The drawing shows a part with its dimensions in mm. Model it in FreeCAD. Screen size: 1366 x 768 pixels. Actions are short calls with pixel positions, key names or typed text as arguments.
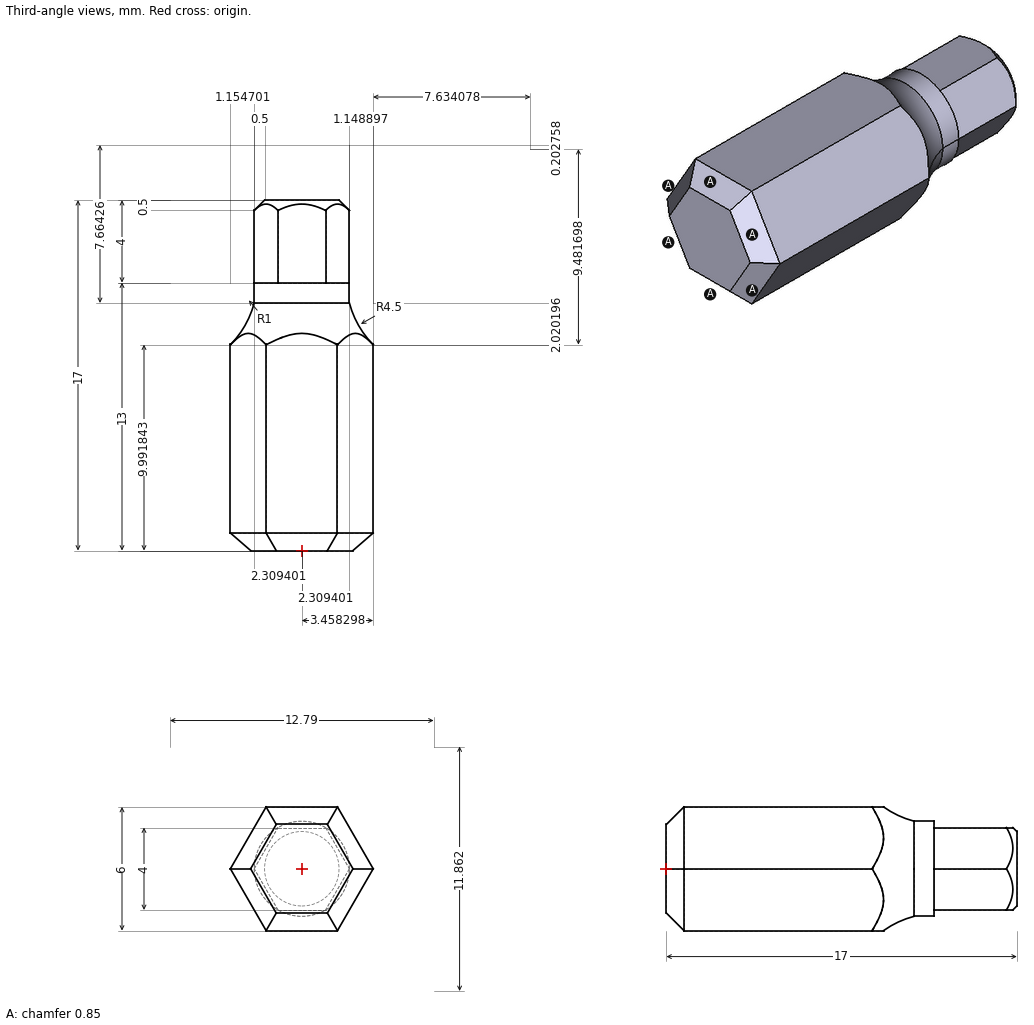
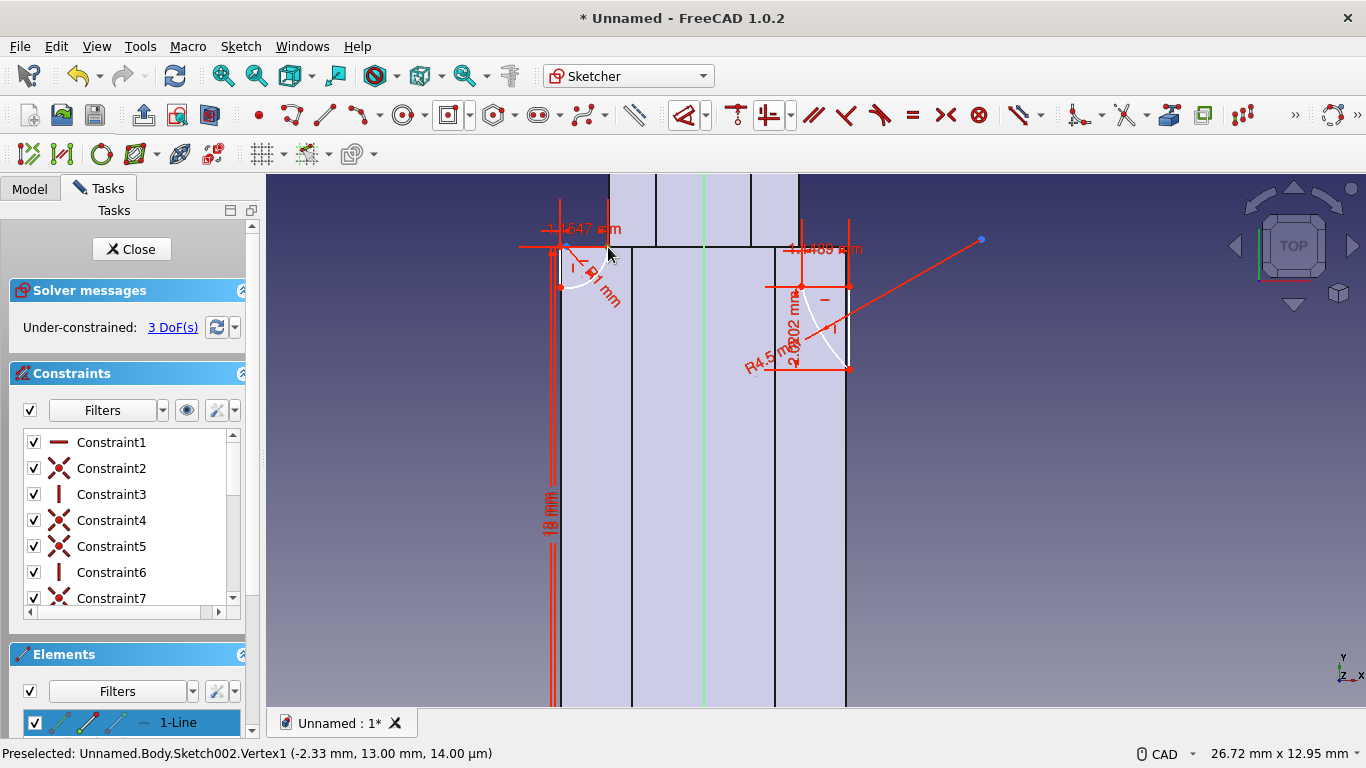
key(l)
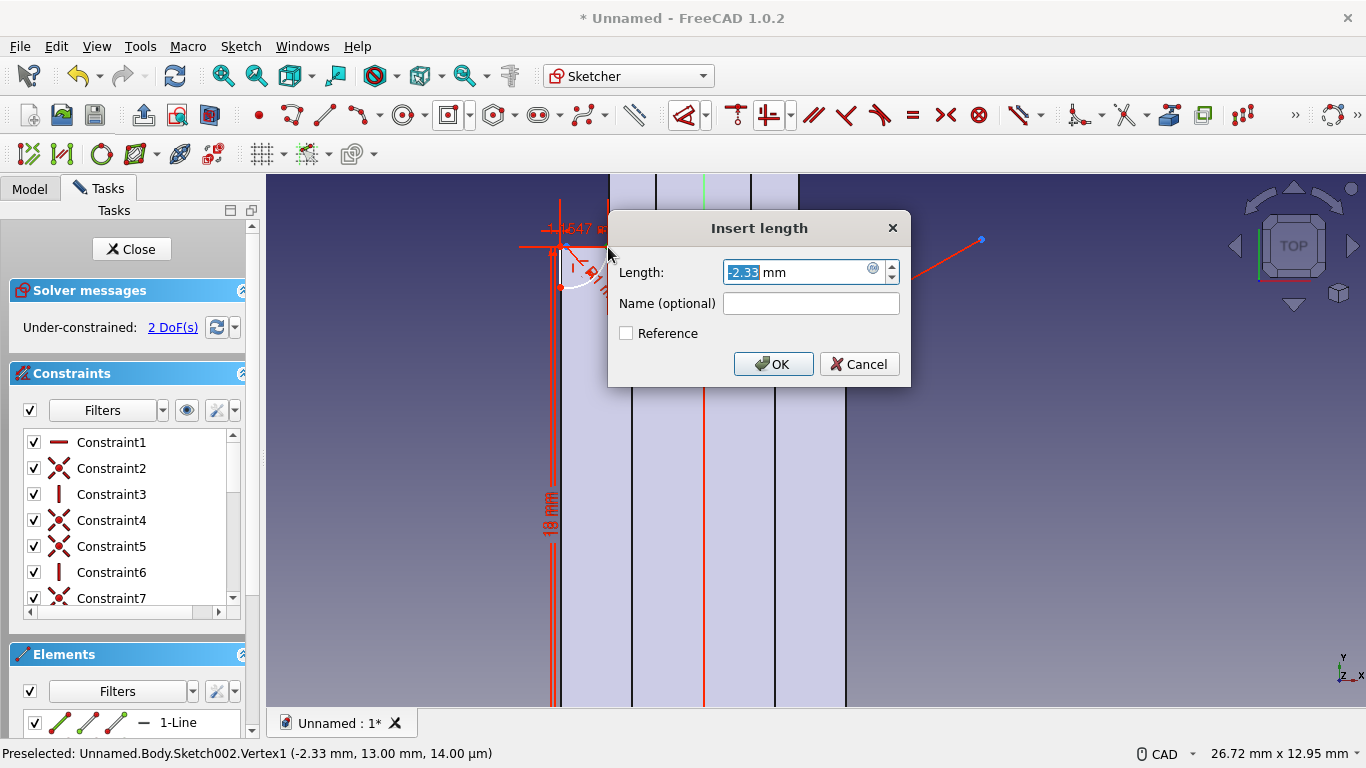
text(-2.309401)
key(Return)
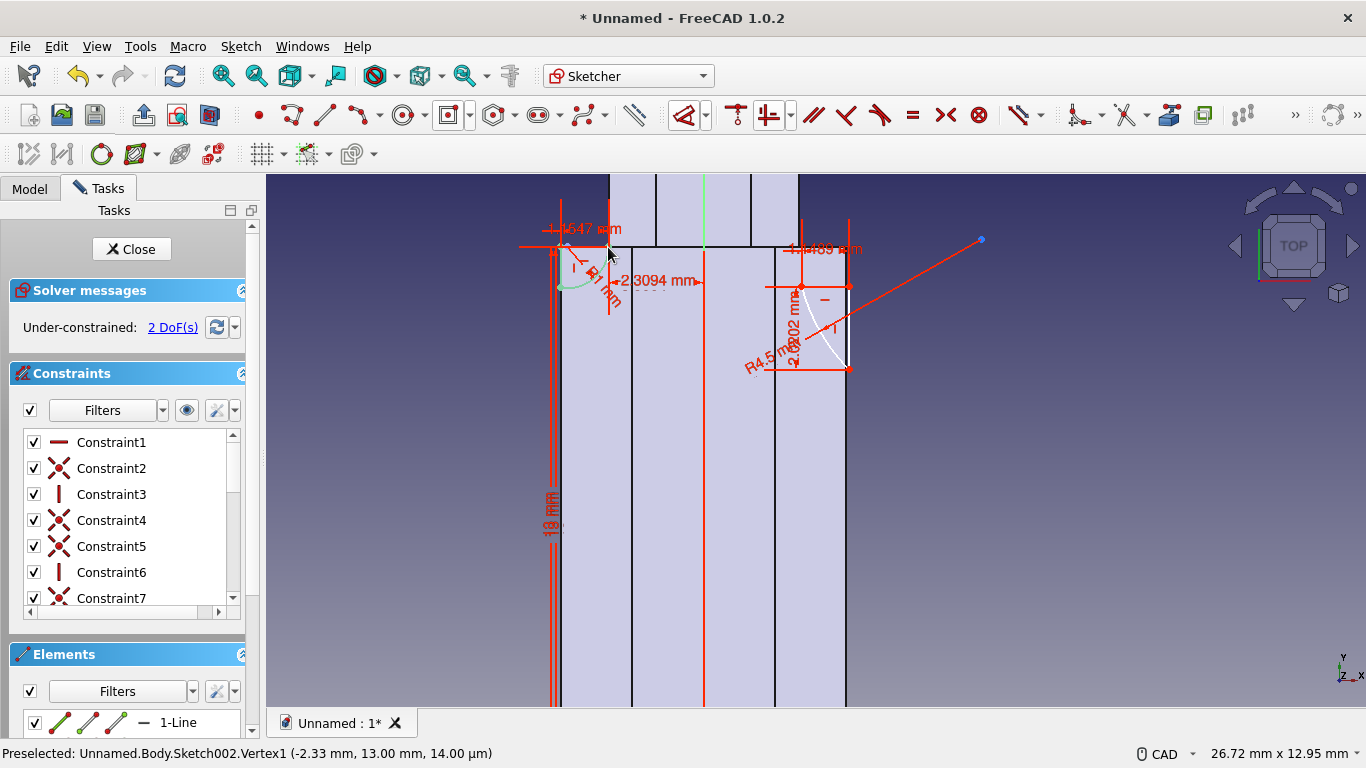
click(849, 370)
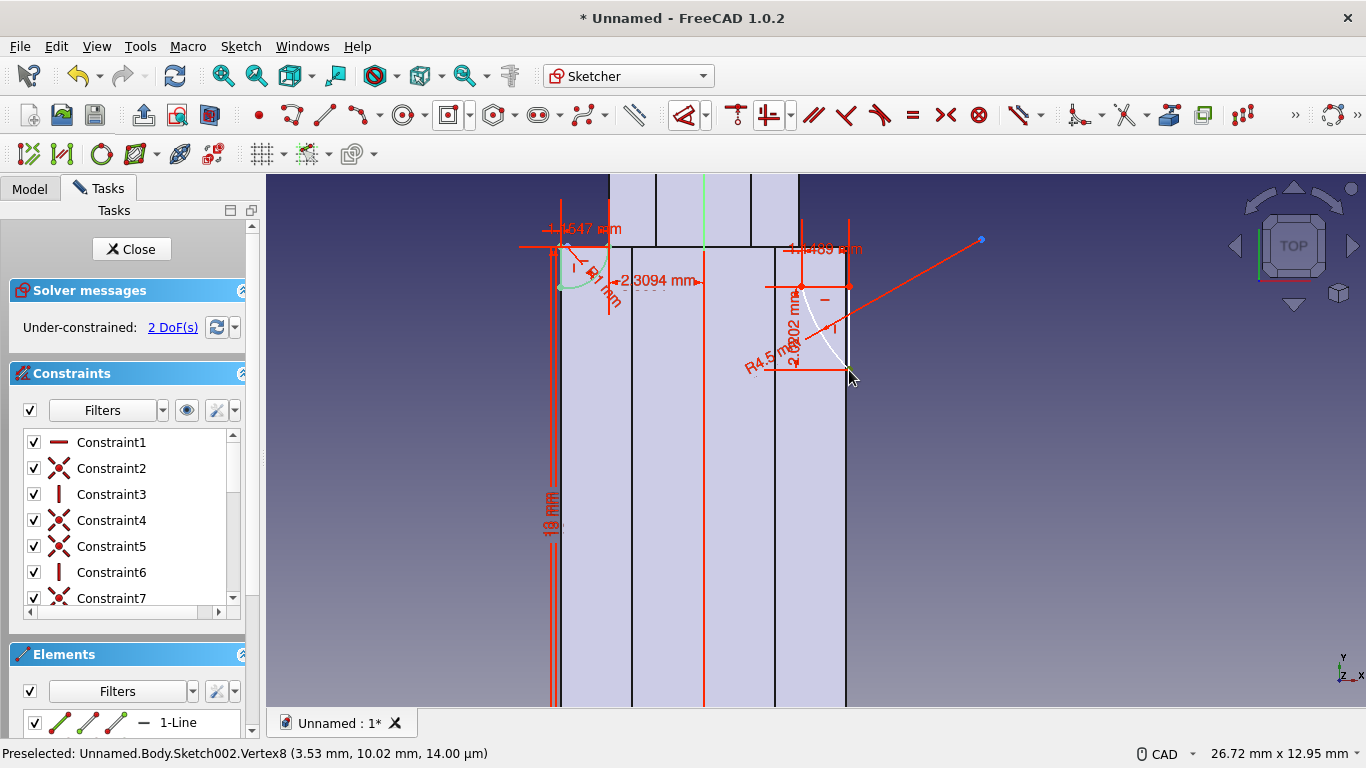
click(706, 116)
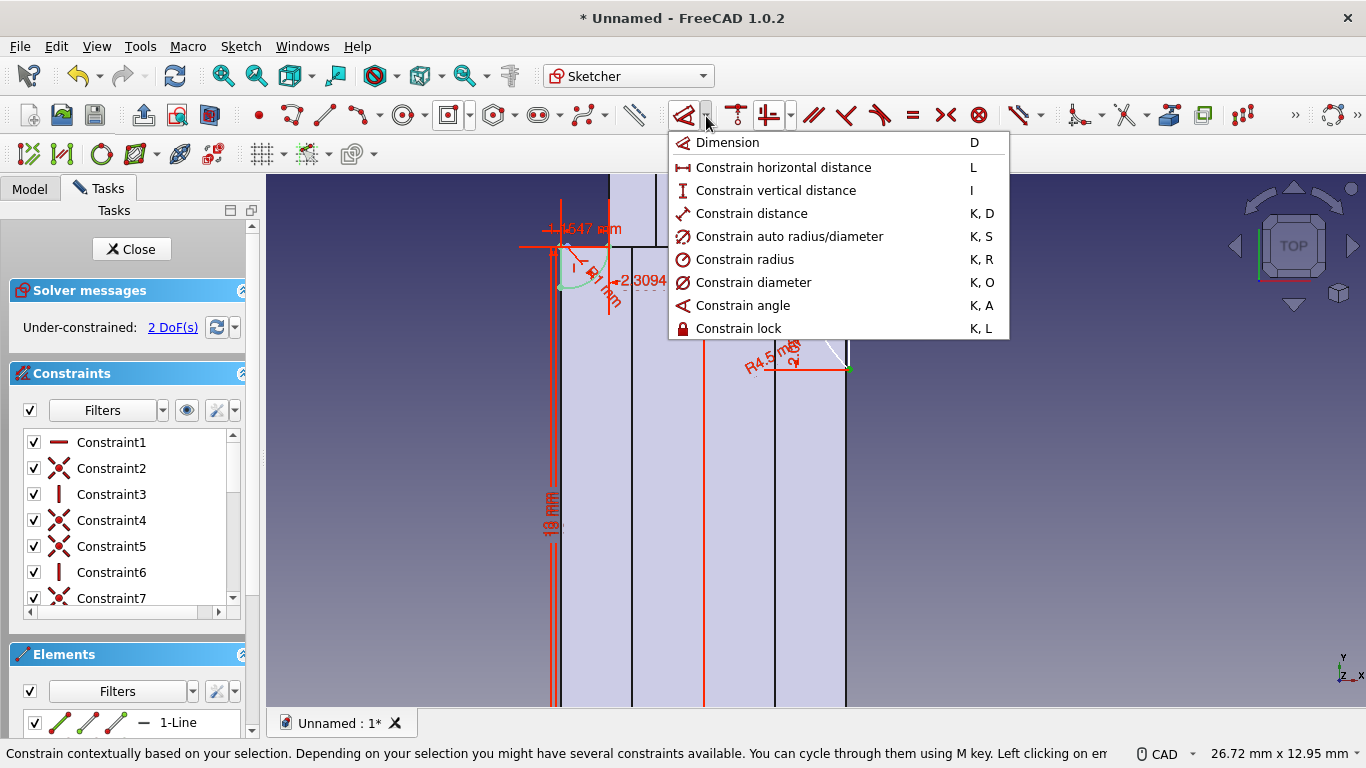
click(839, 168)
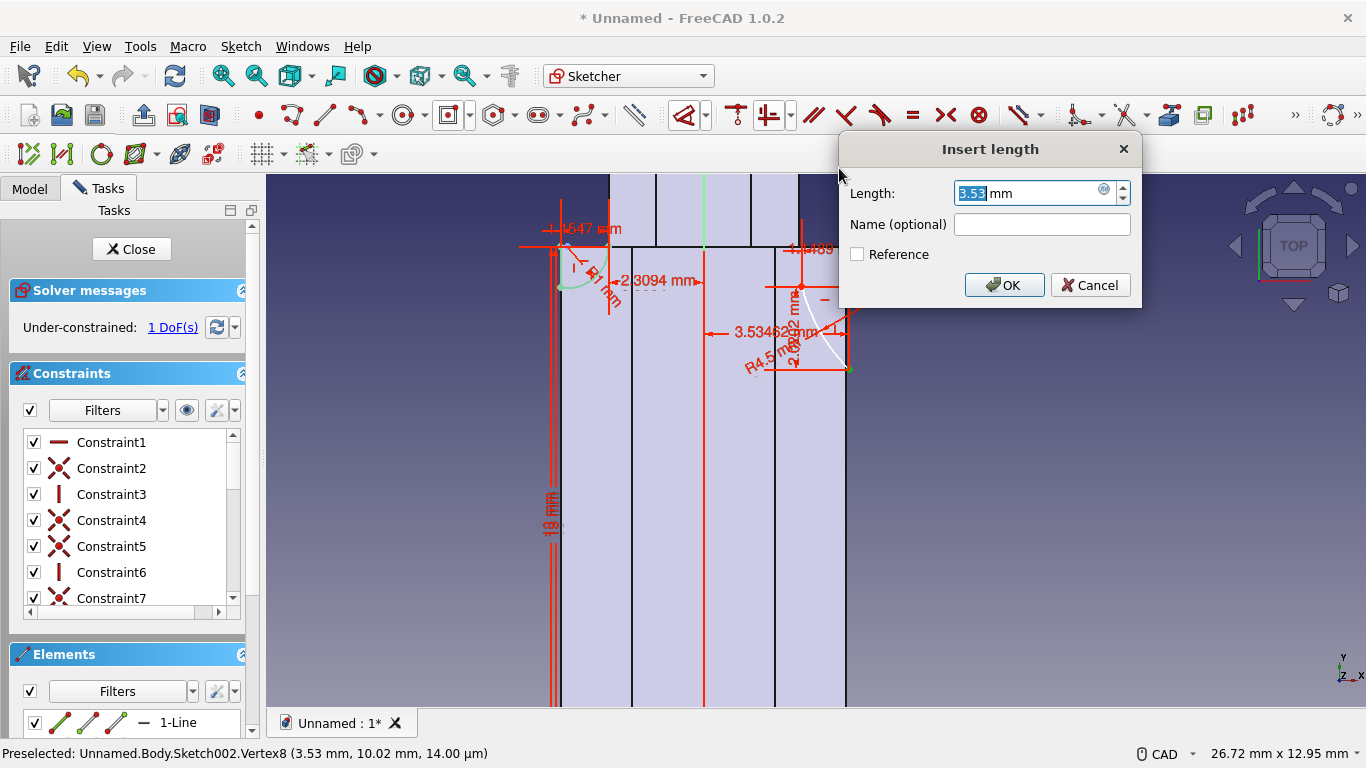
text(3.458298)
key(Return)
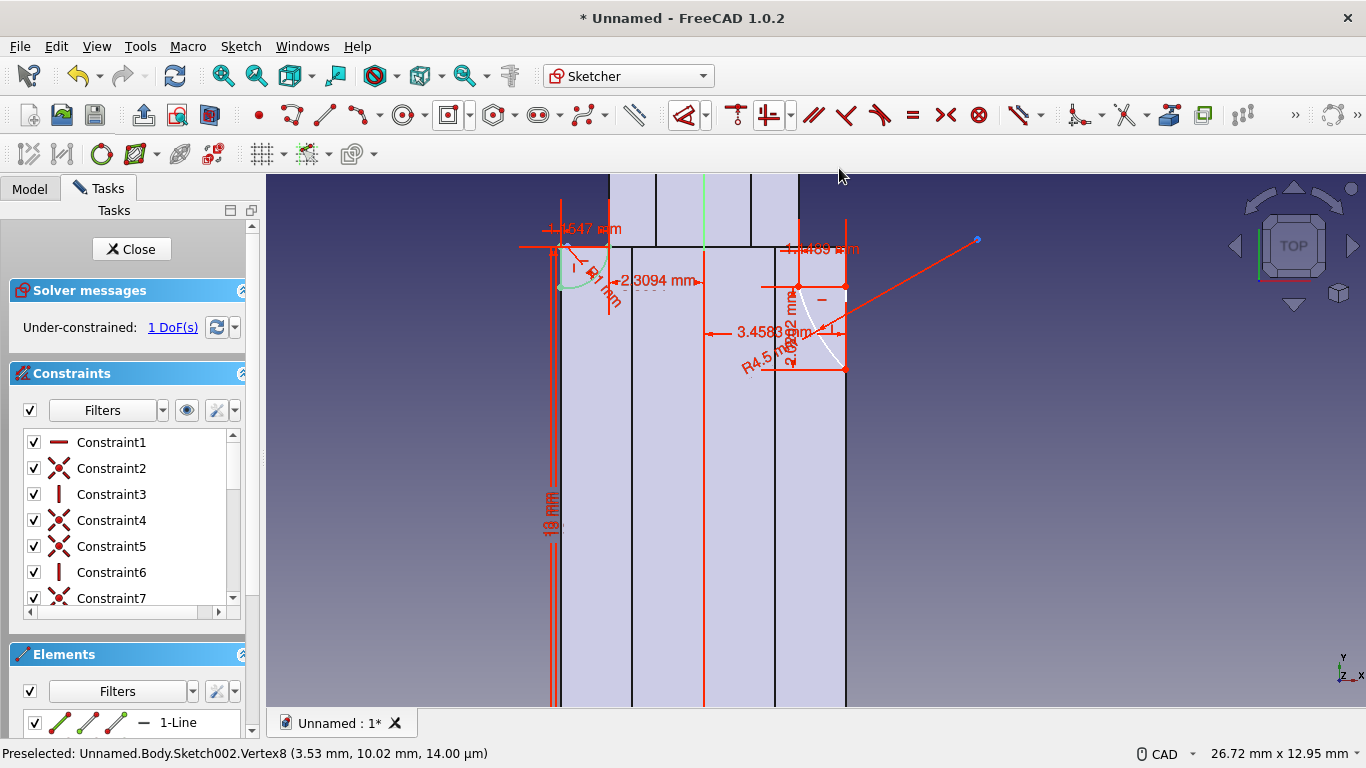
click(846, 370)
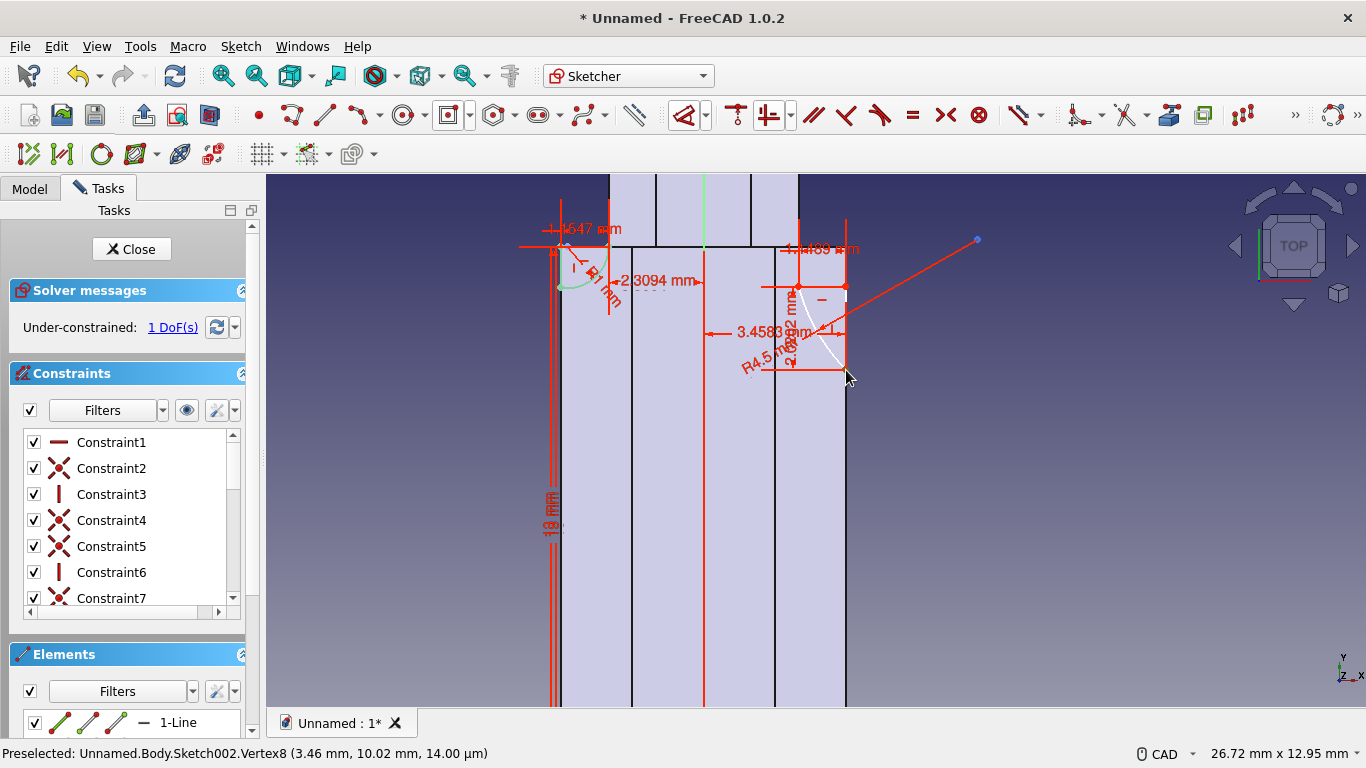
key(i)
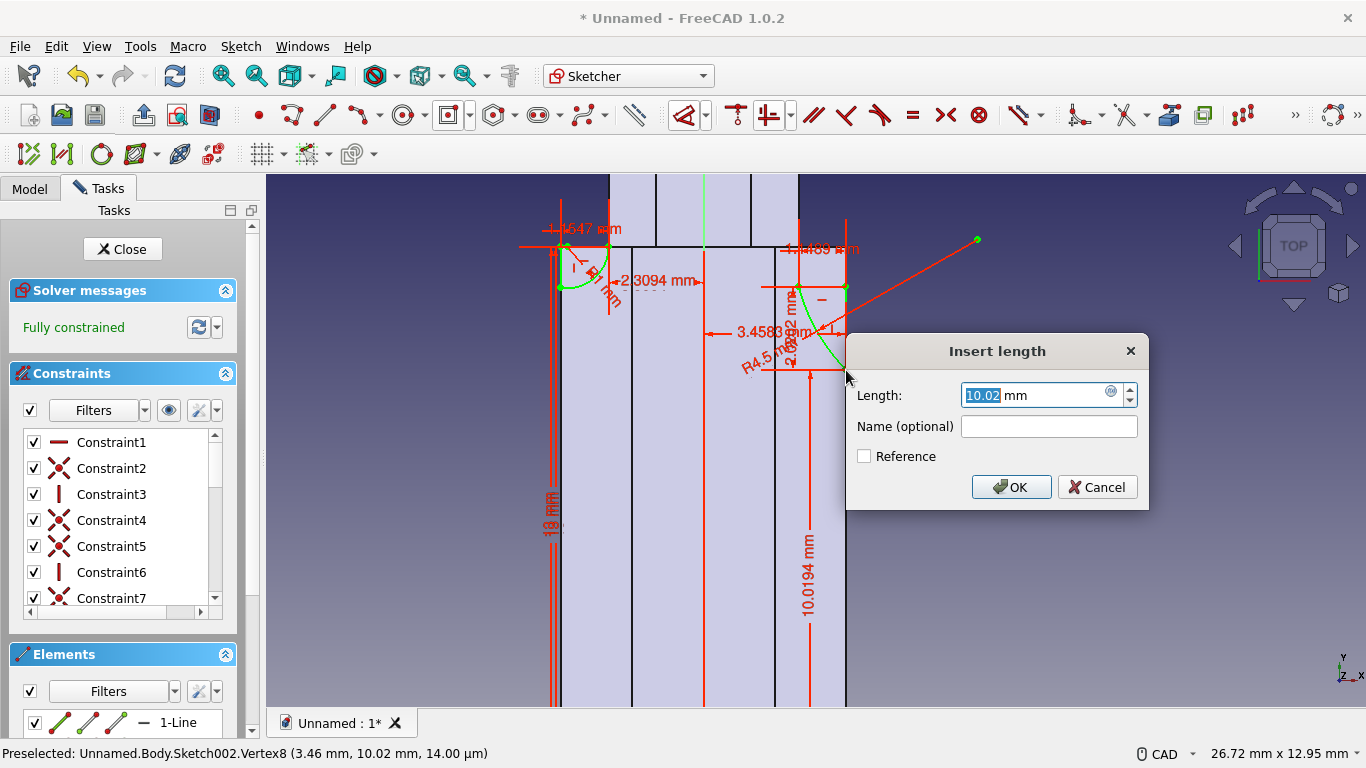
text(9.991843)
key(Return)